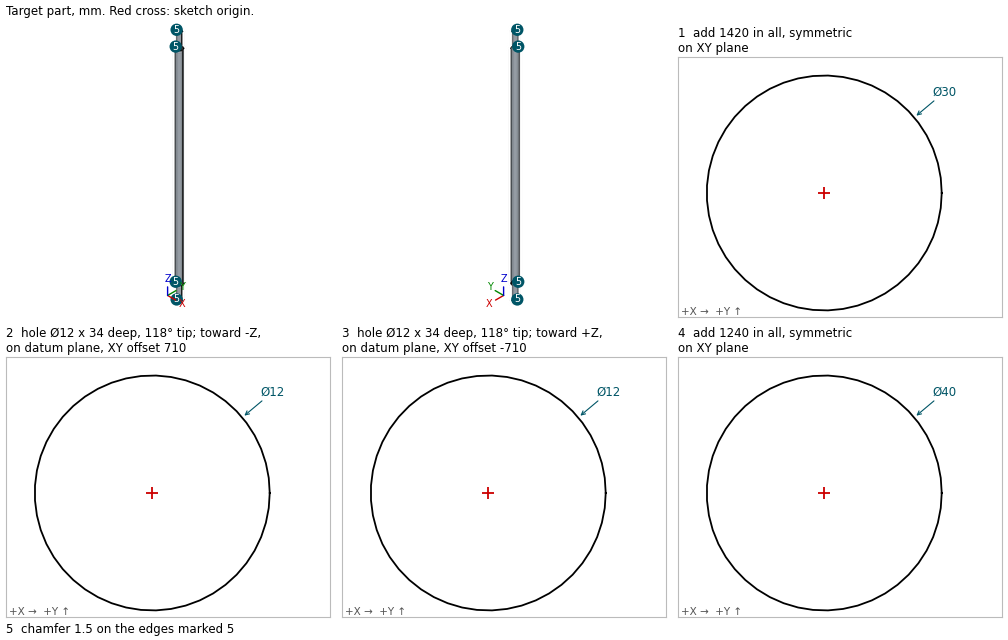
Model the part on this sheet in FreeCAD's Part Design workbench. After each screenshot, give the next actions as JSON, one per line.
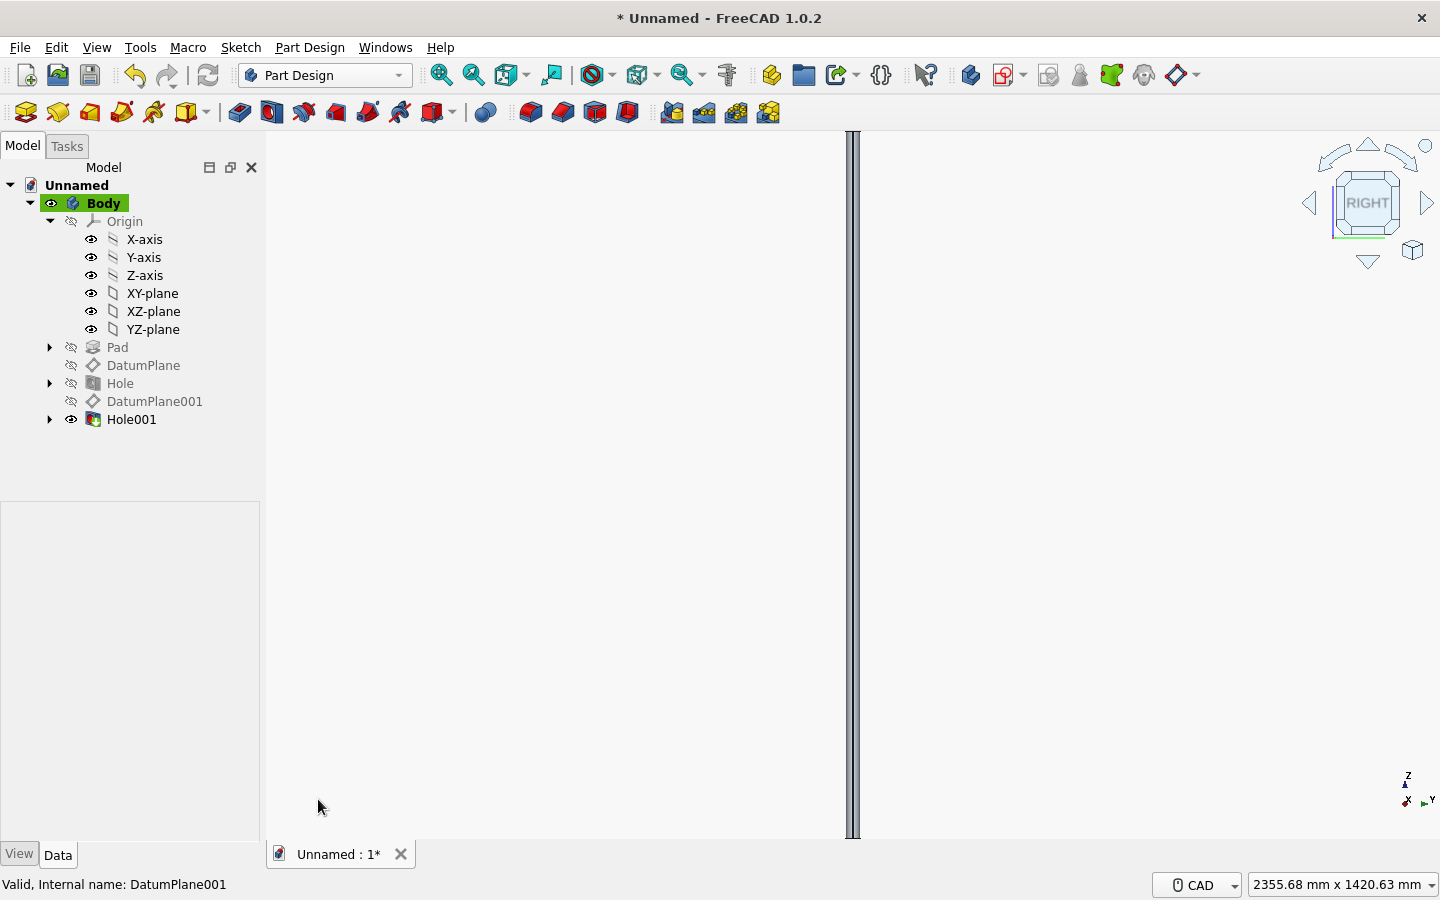
{"action": "left_click", "coordinate": [1004, 76]}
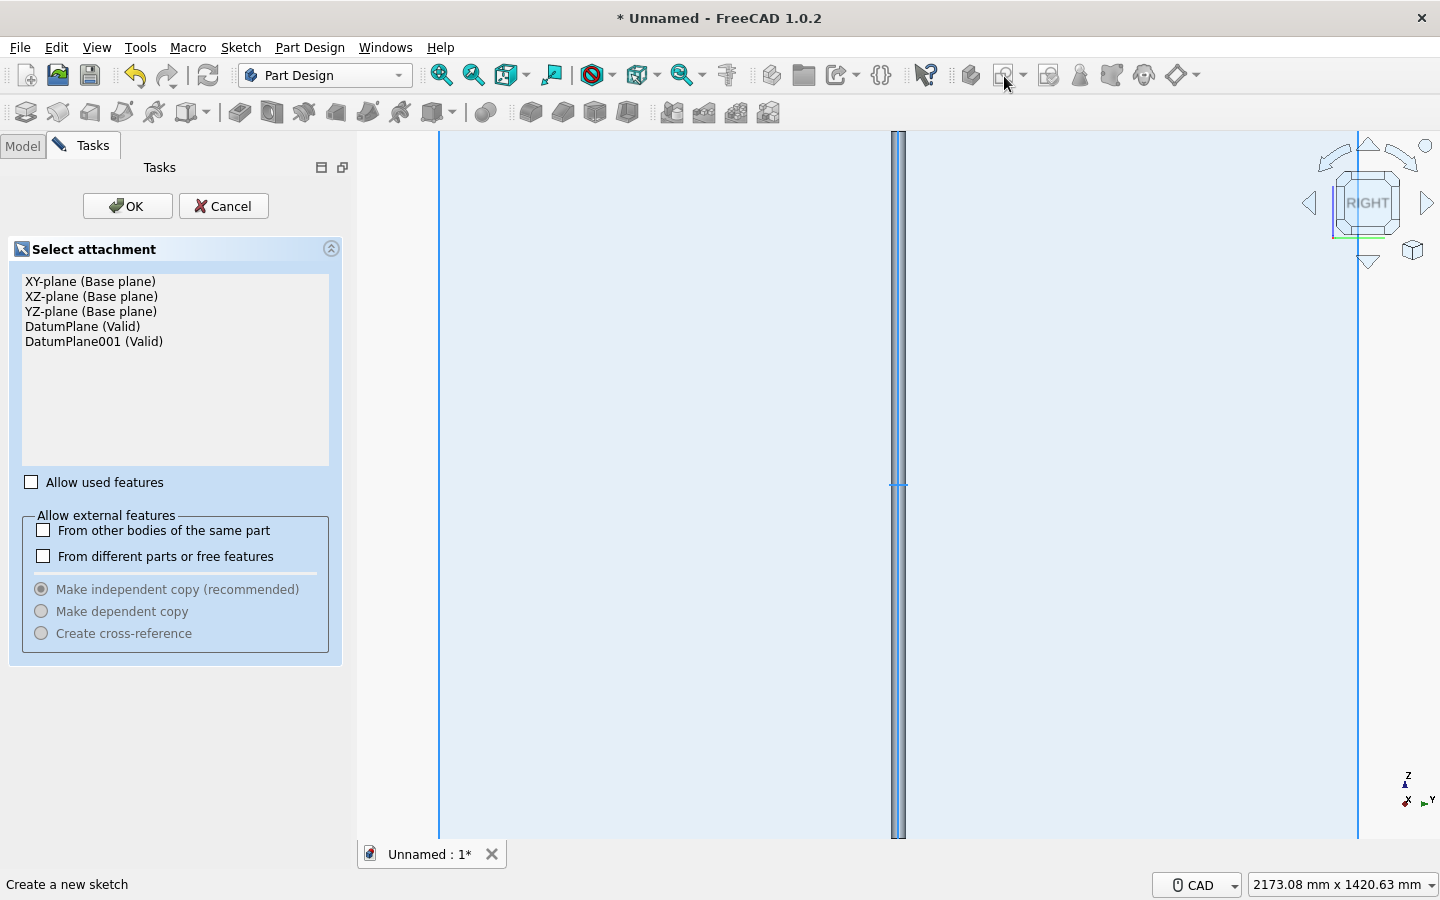
{"action": "left_click", "coordinate": [82, 282]}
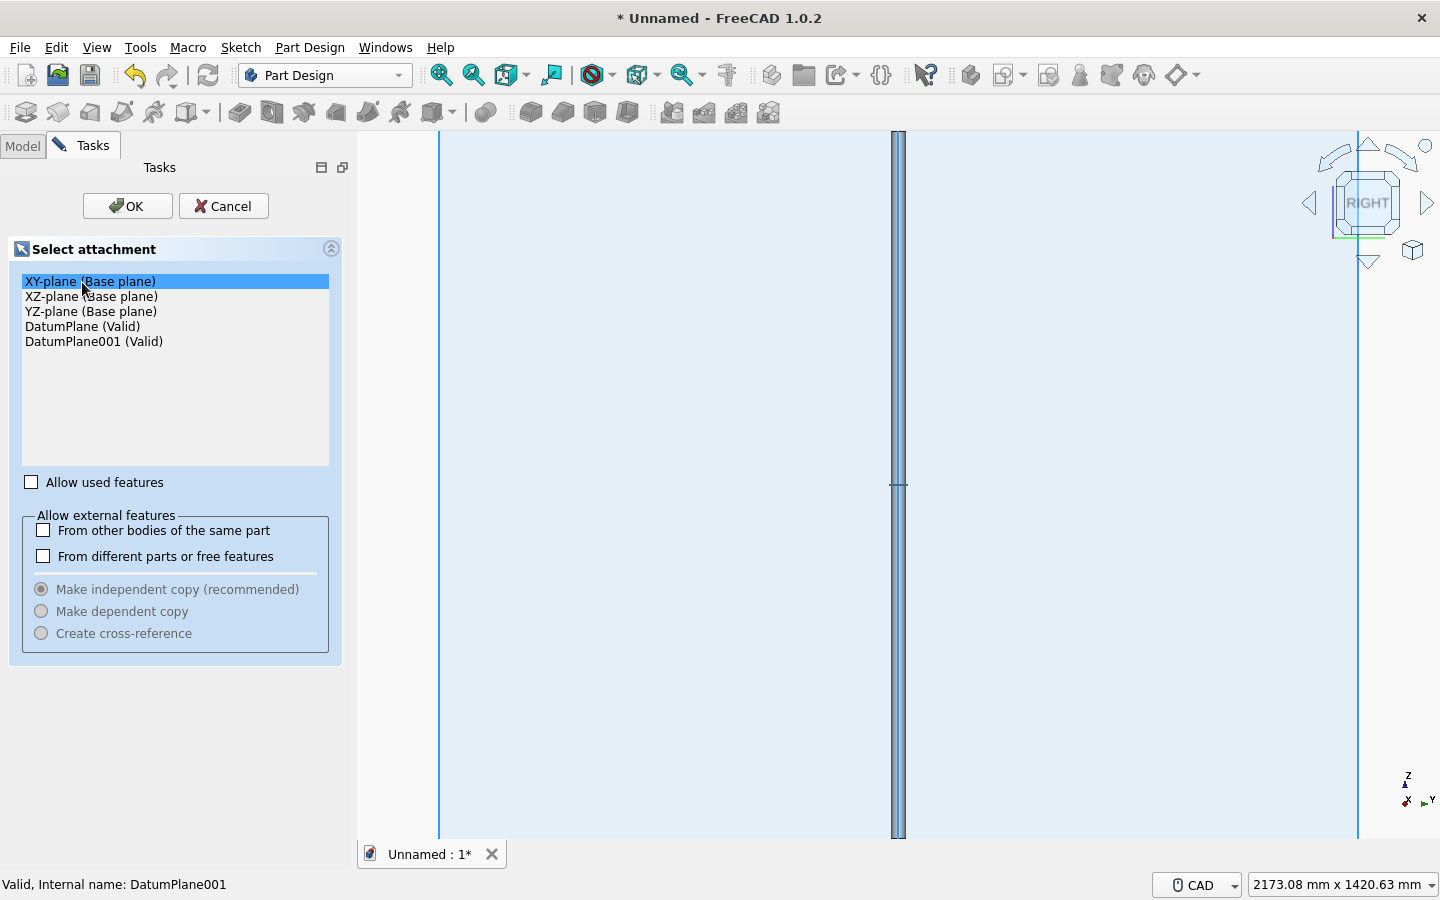
{"action": "left_click", "coordinate": [128, 206]}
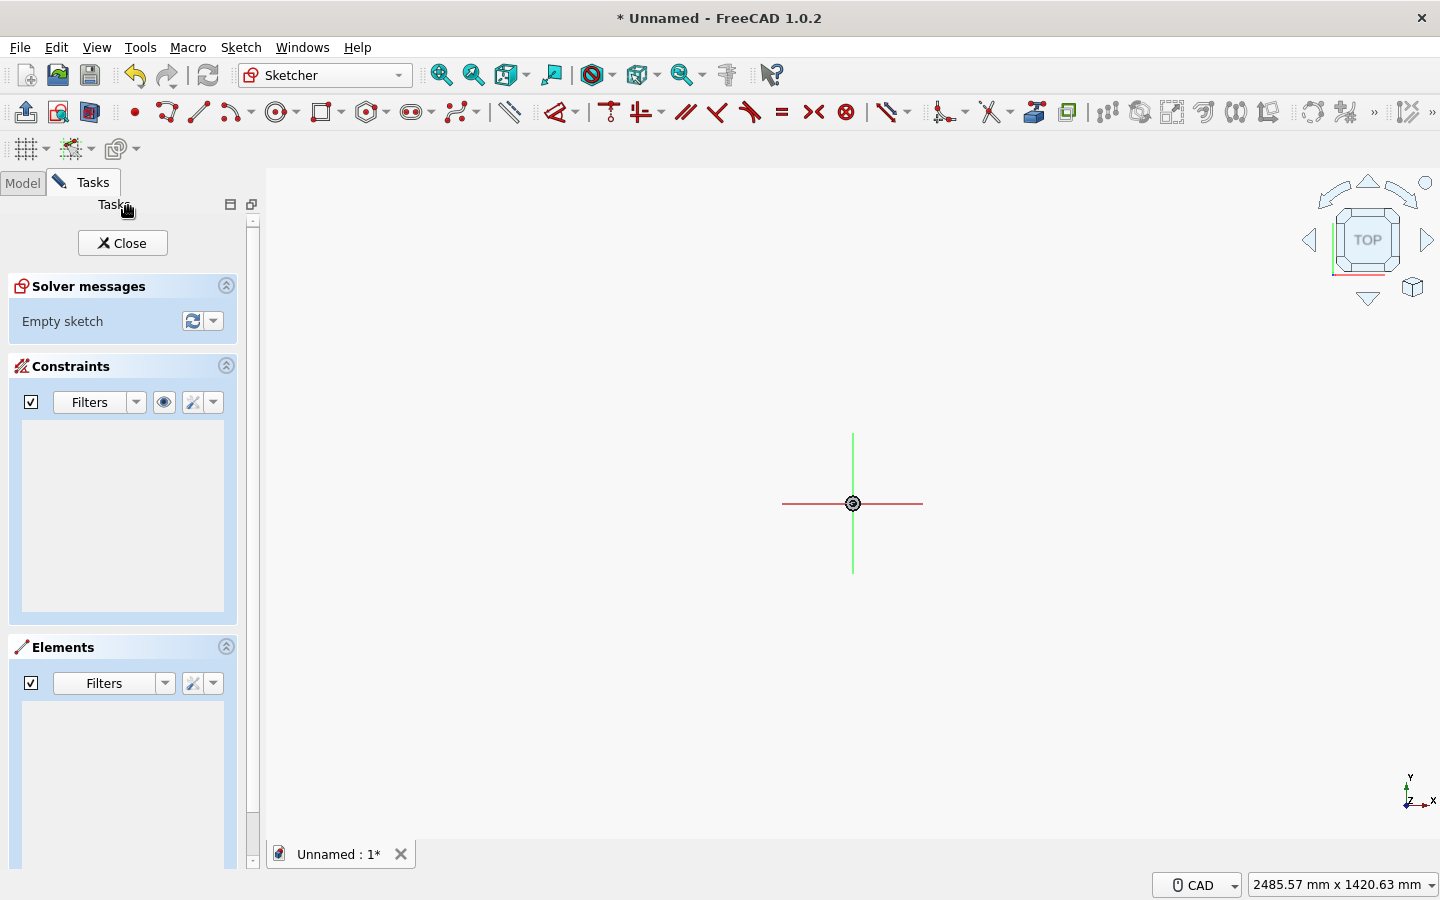
{"action": "left_click", "coordinate": [90, 112]}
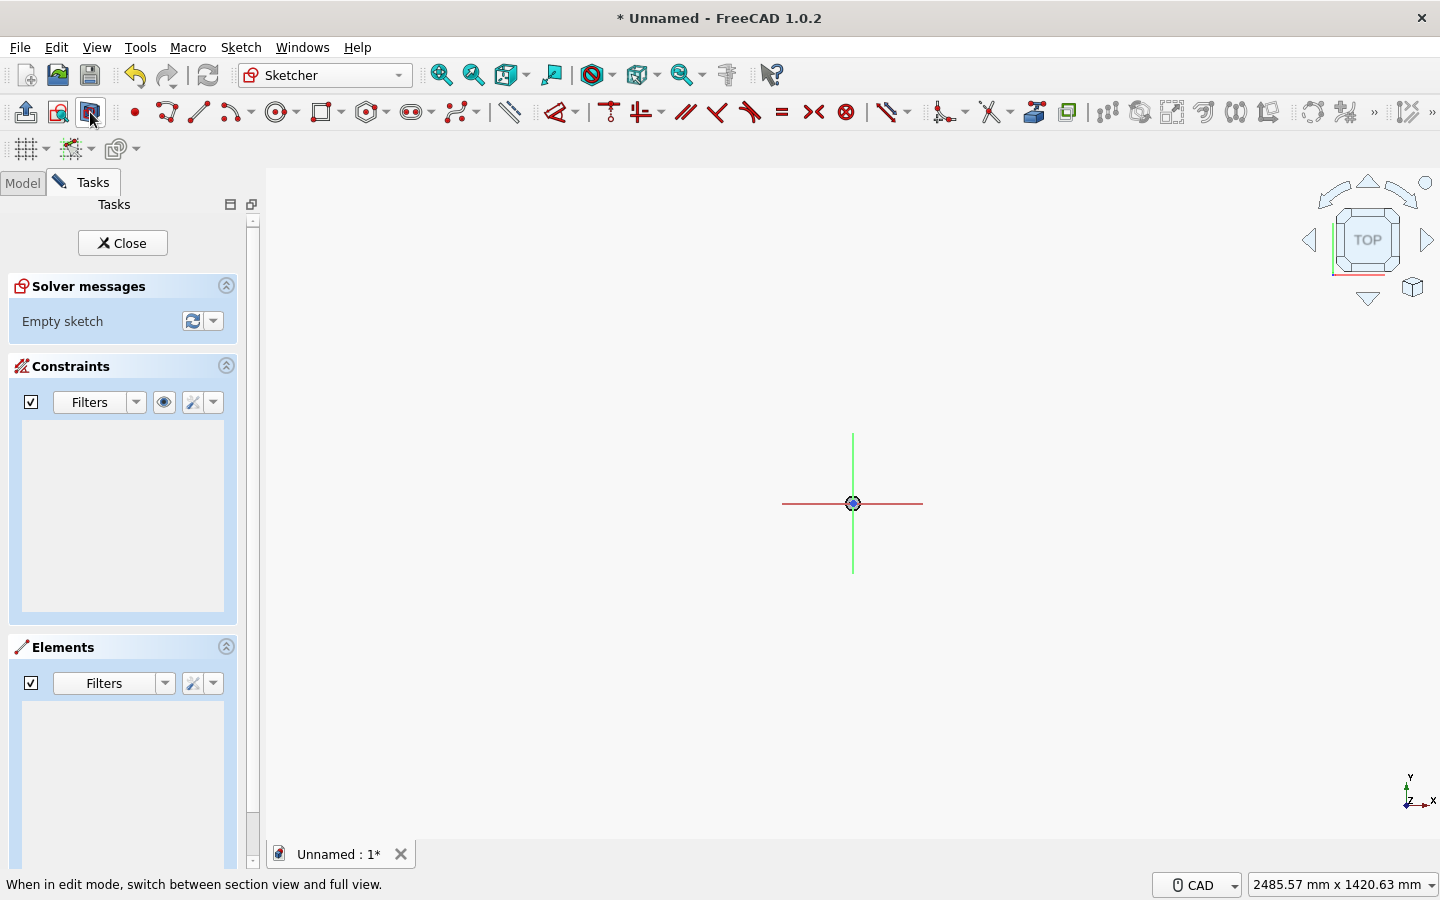
{"action": "scroll", "coordinate": [857, 504], "scroll_direction": "up", "scroll_amount": 15}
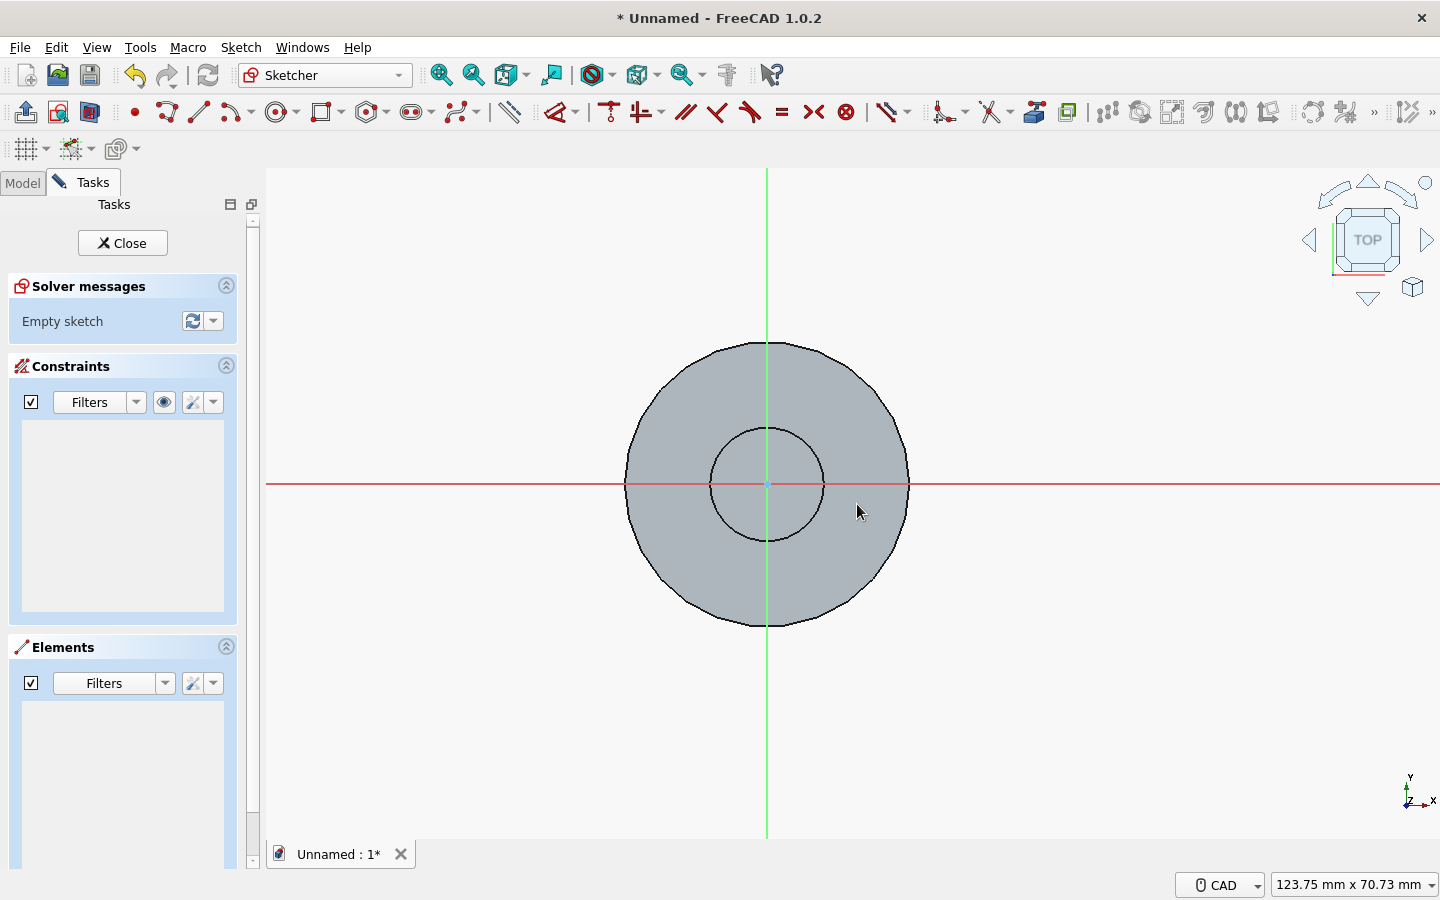
{"action": "left_click", "coordinate": [276, 112]}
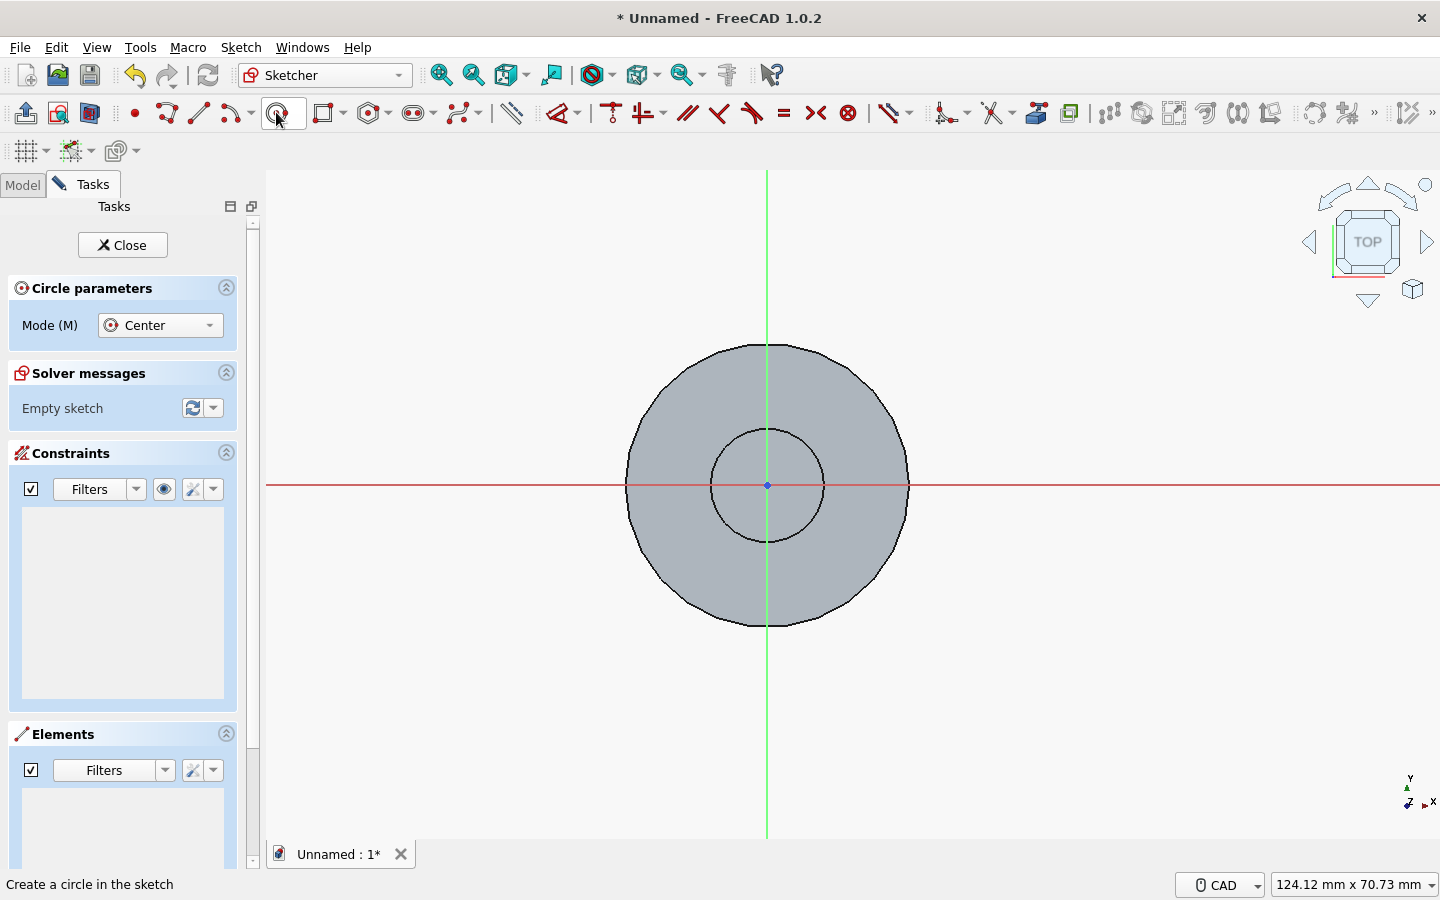
{"action": "left_click", "coordinate": [767, 485]}
{"action": "mouse_move", "coordinate": [901, 352]}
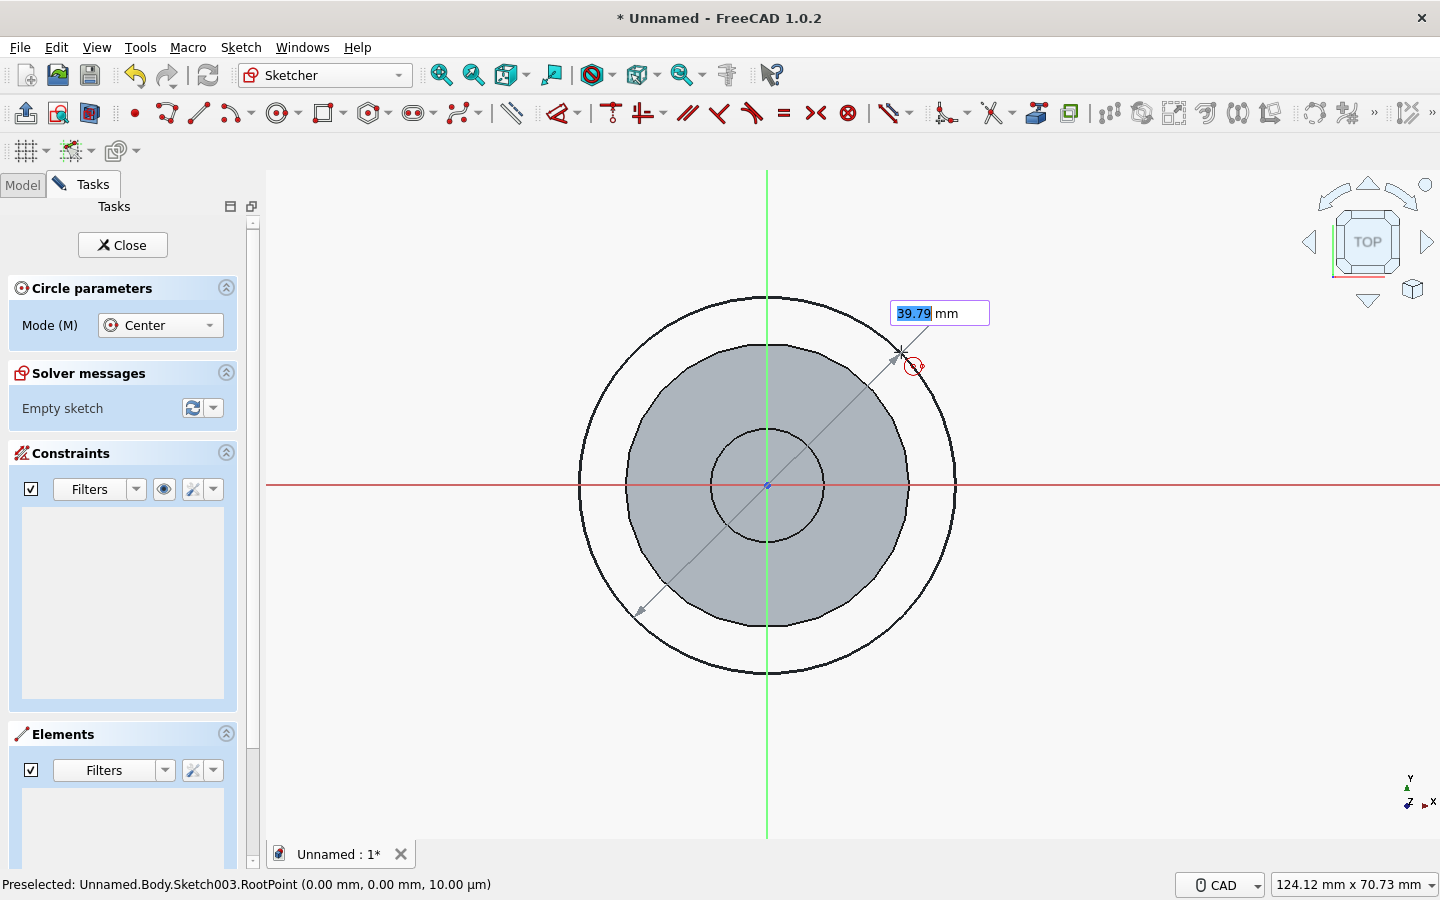
{"action": "type", "text": "40"}
{"action": "key", "text": "Return"}
{"action": "key", "text": "Escape"}